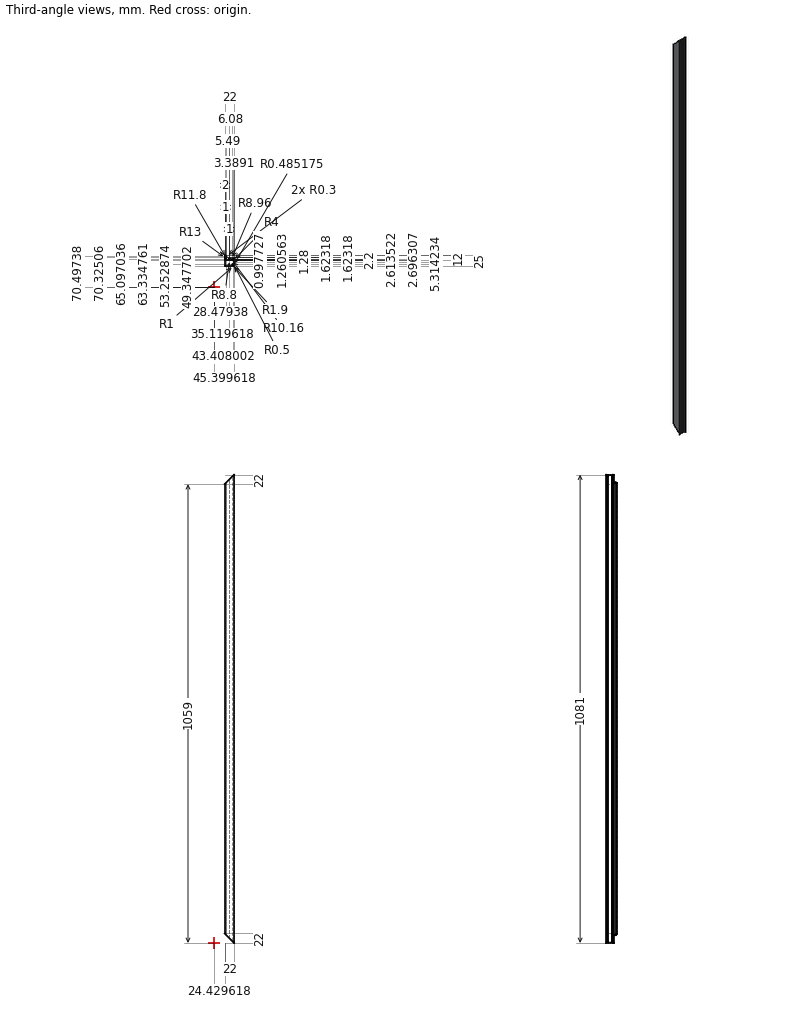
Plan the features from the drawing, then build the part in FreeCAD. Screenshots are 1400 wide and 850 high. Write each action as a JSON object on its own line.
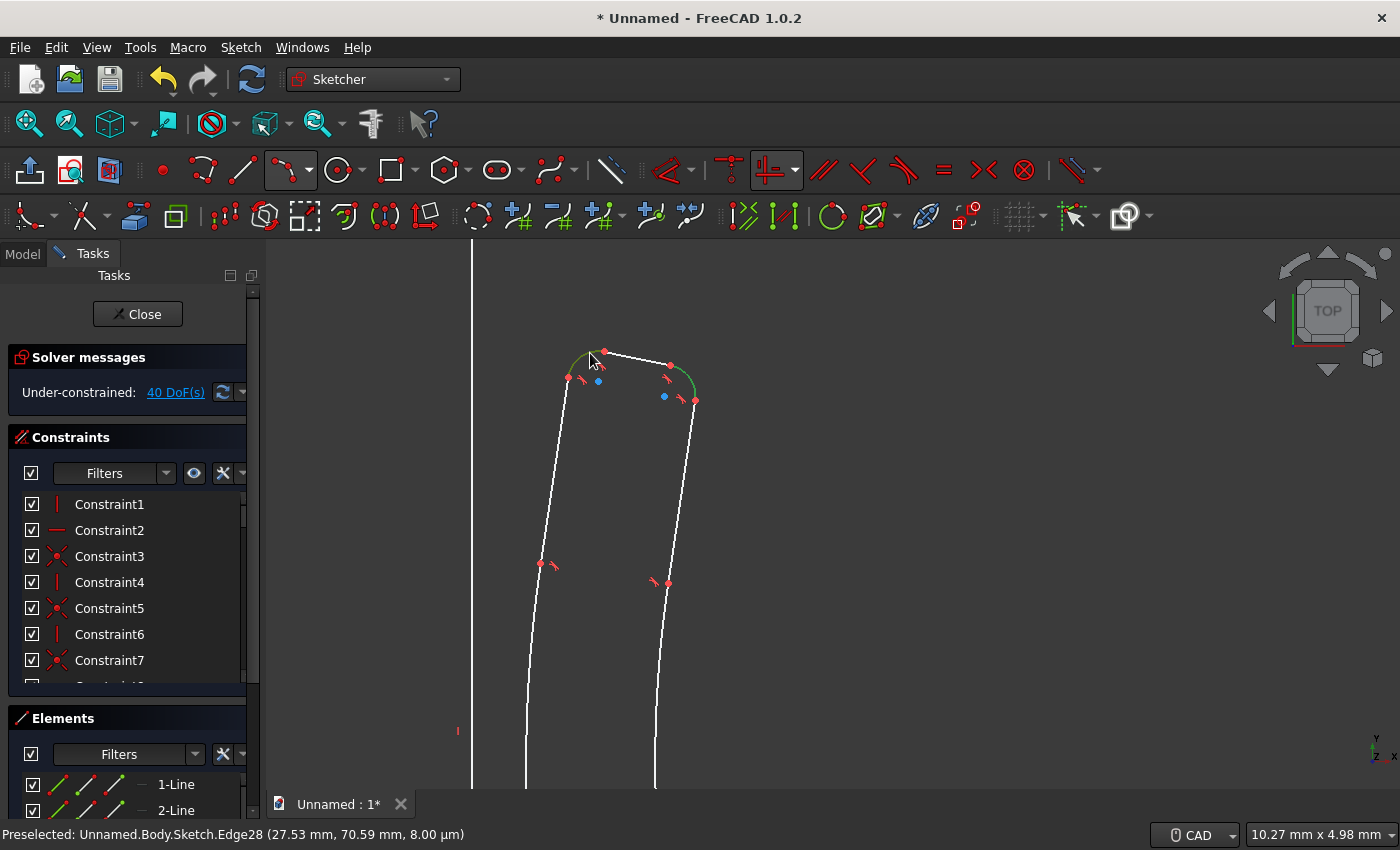
{"action": "left_click", "coordinate": [944, 170]}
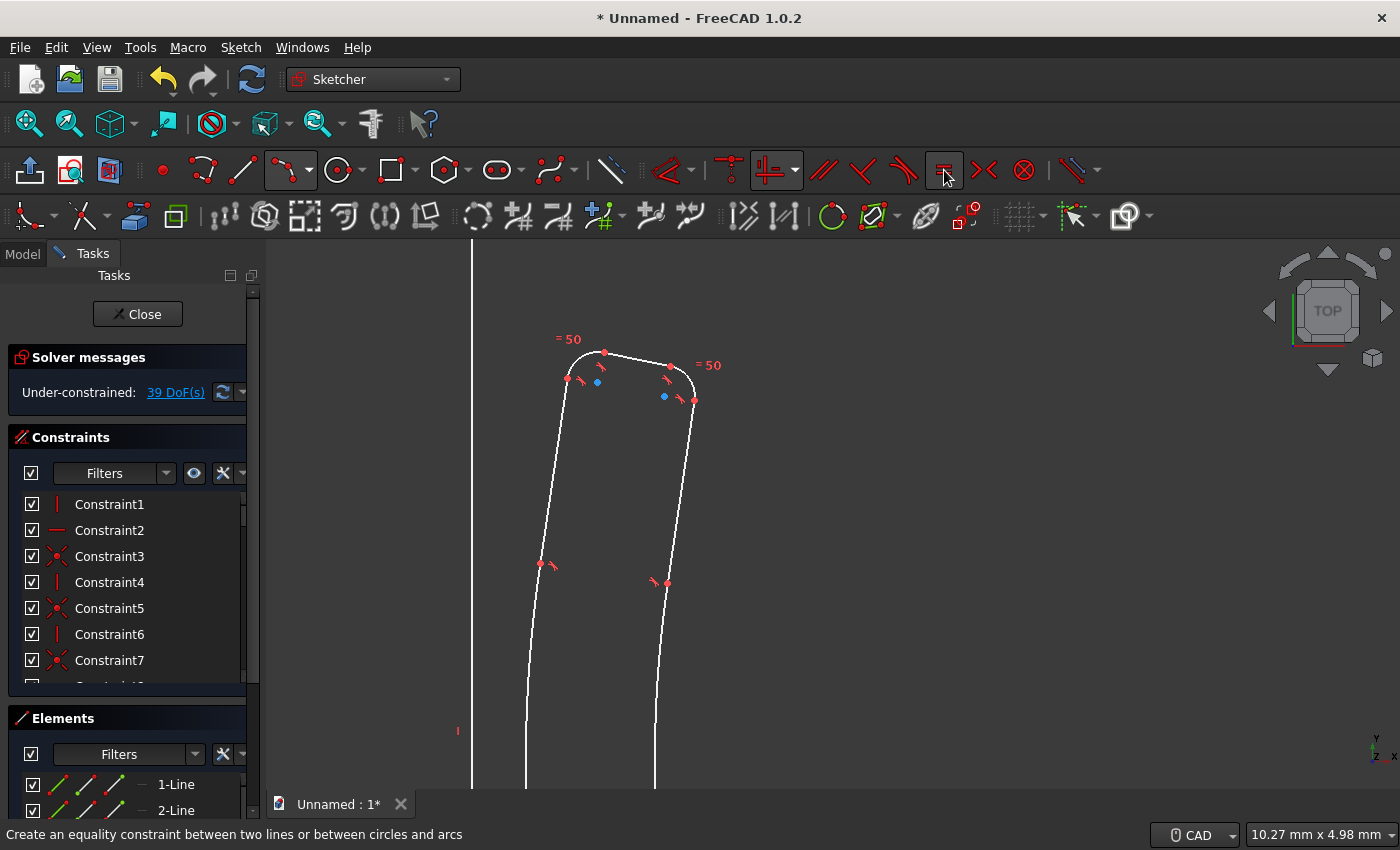
{"action": "scroll", "coordinate": [655, 368], "scroll_direction": "down", "scroll_amount": 10}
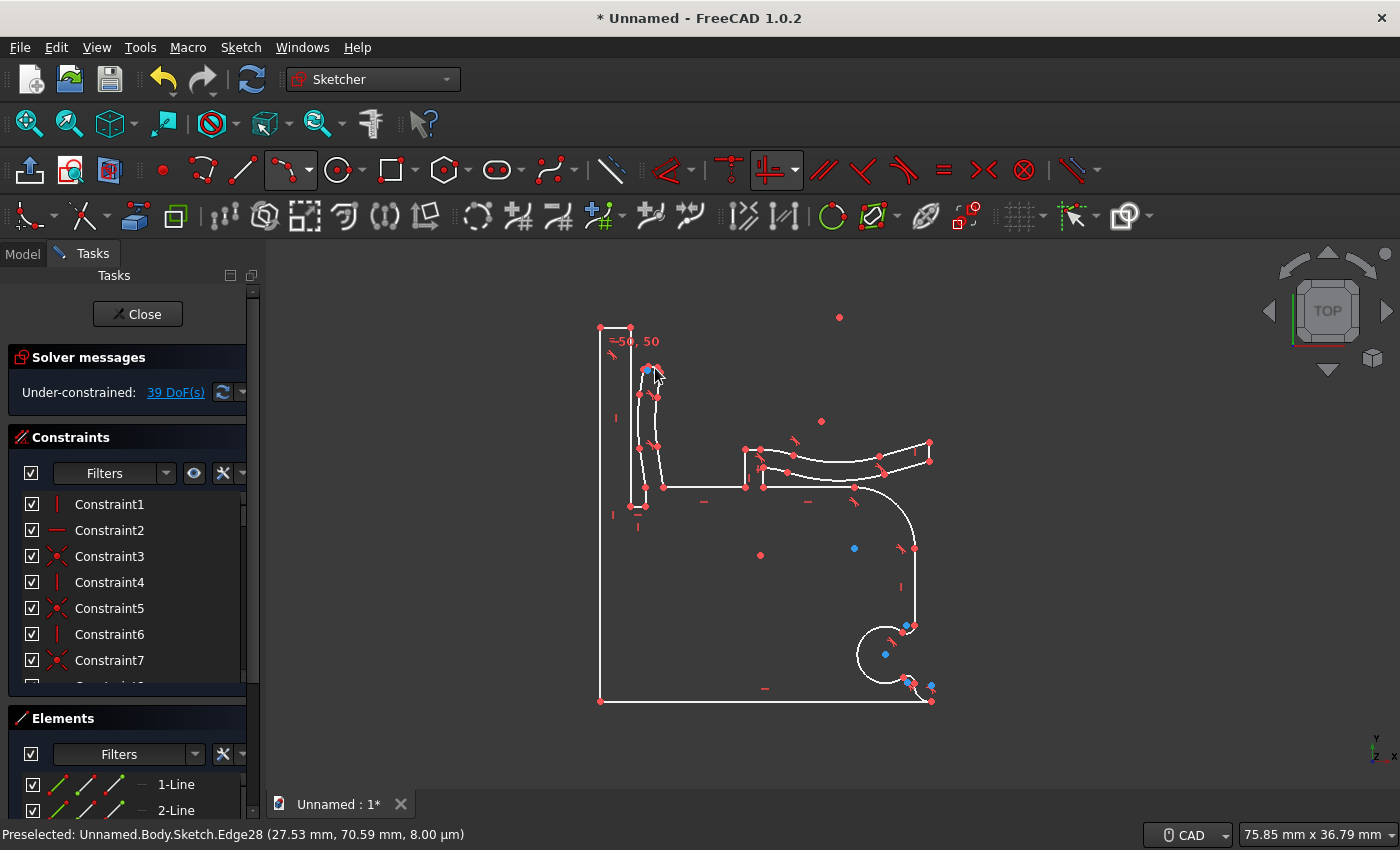
{"action": "left_click", "coordinate": [908, 521]}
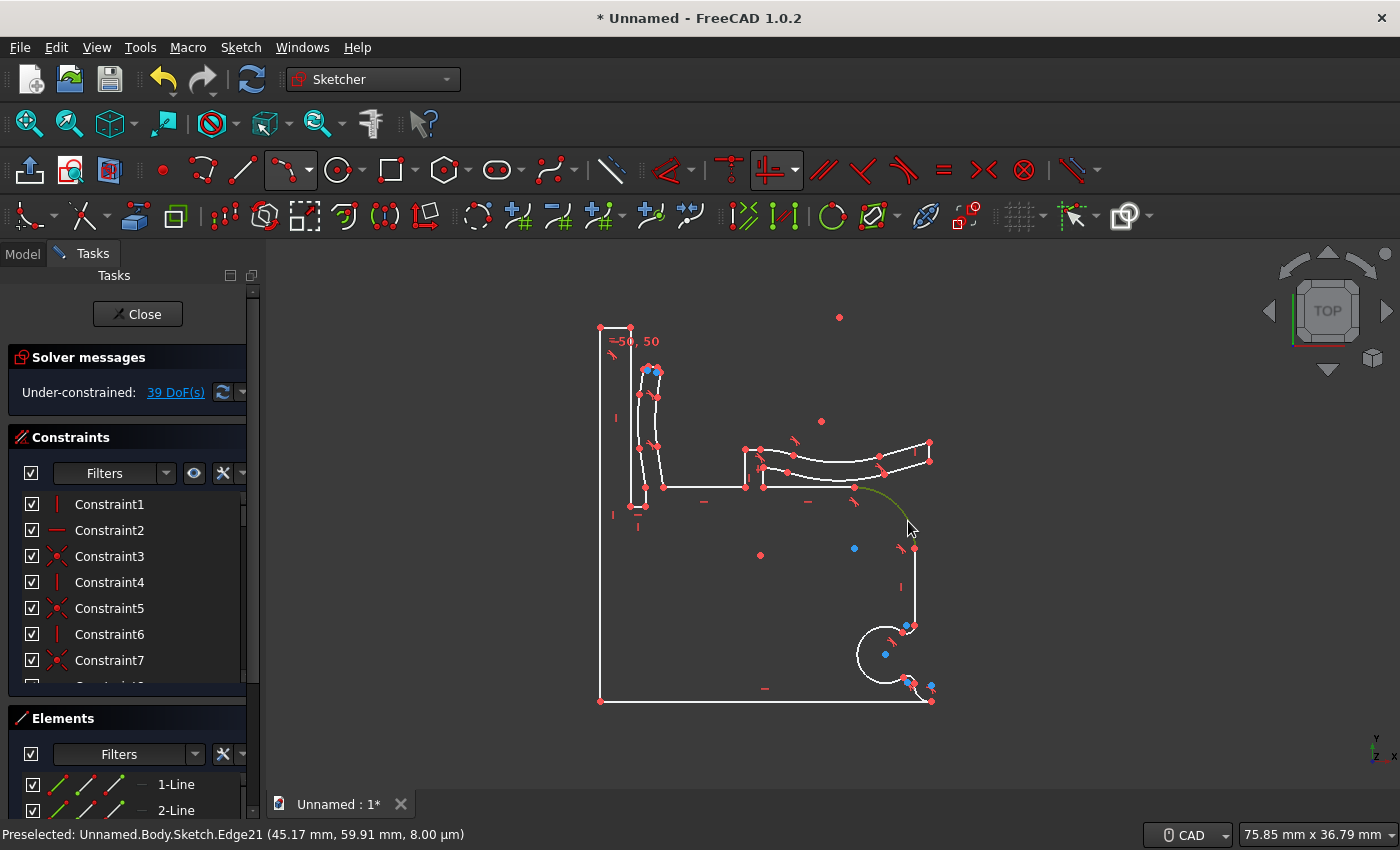
{"action": "key", "text": "k r"}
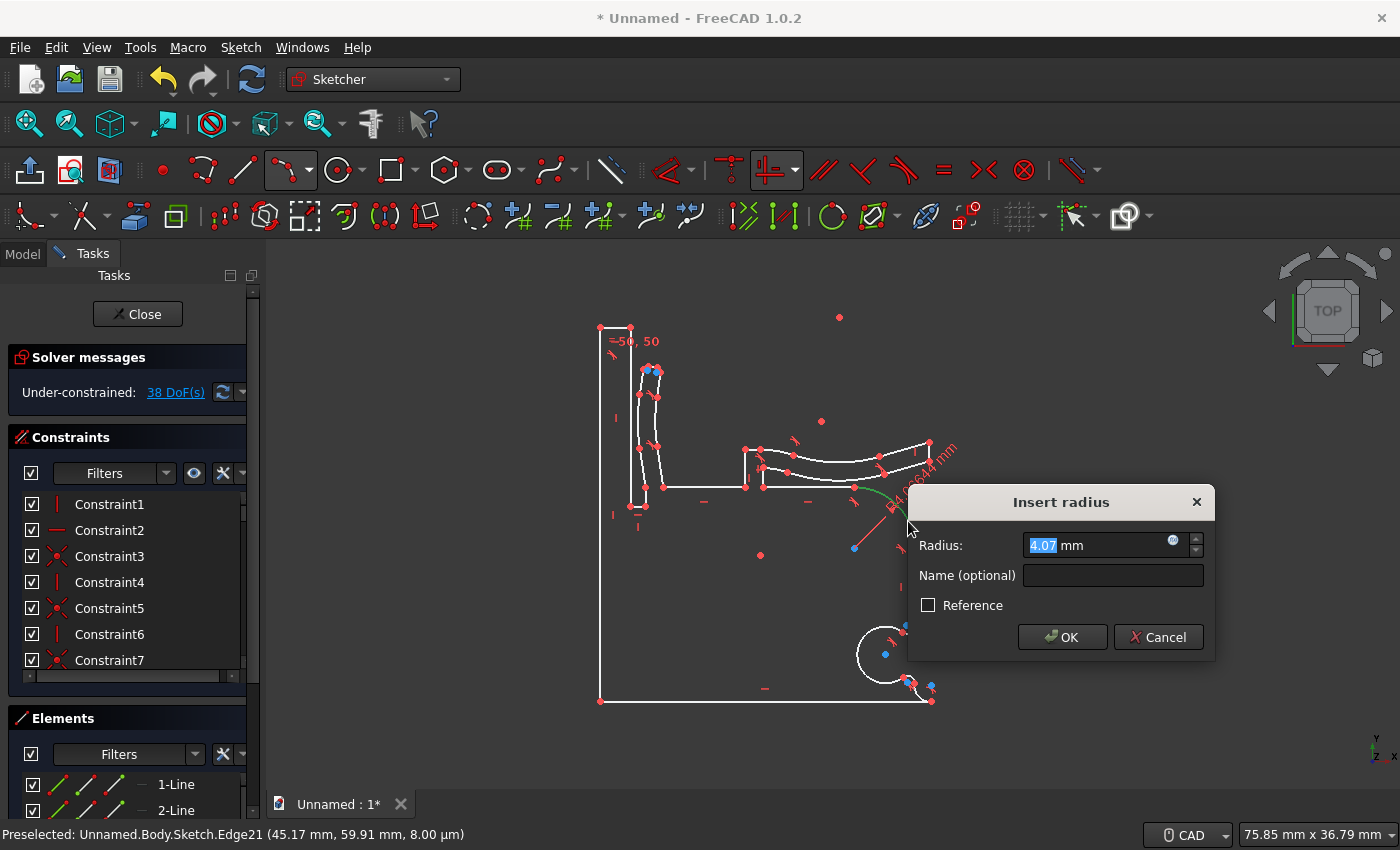
{"action": "type", "text": "4"}
{"action": "key", "text": "Return"}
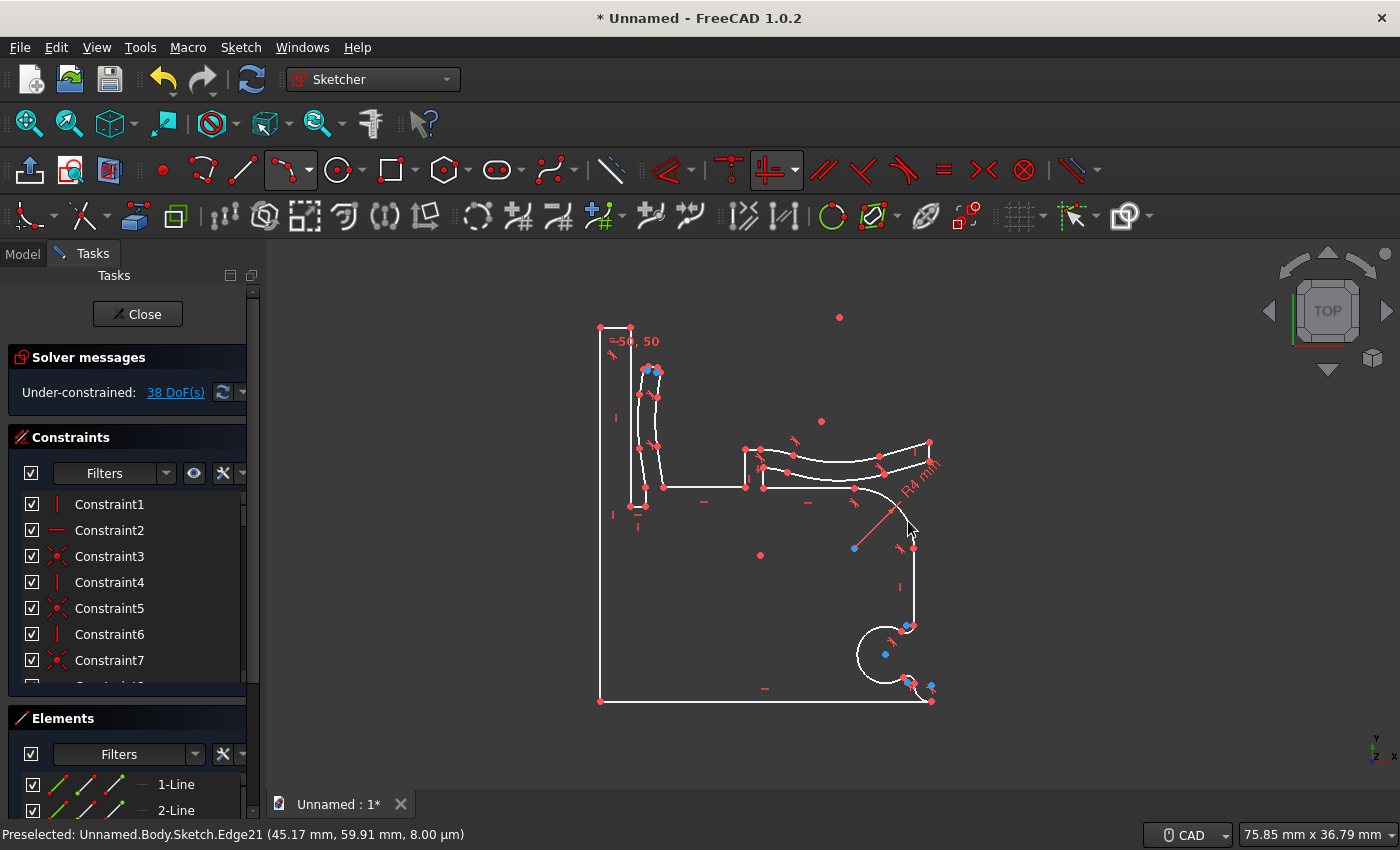
{"action": "left_click", "coordinate": [776, 469]}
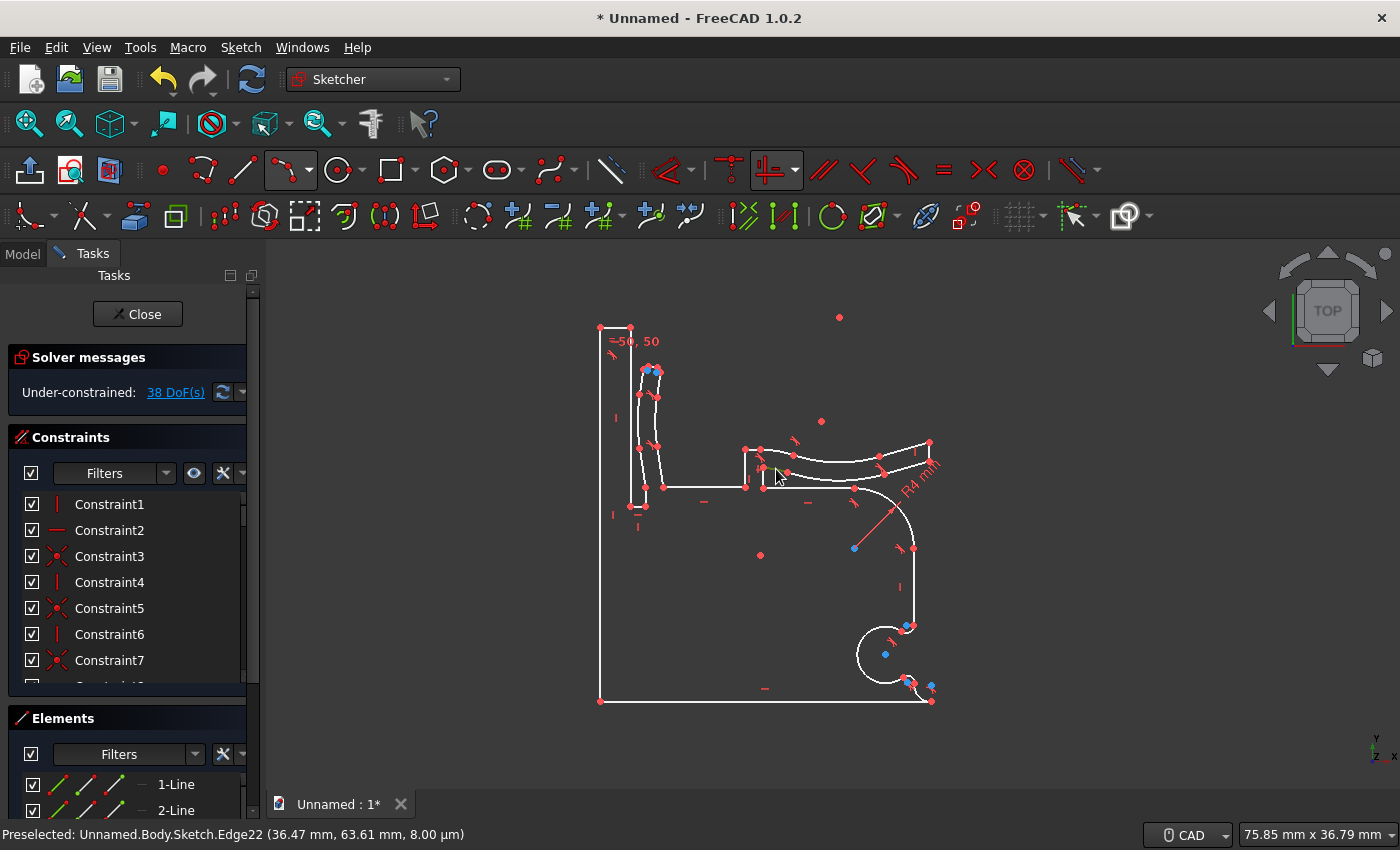
{"action": "key", "text": "k r"}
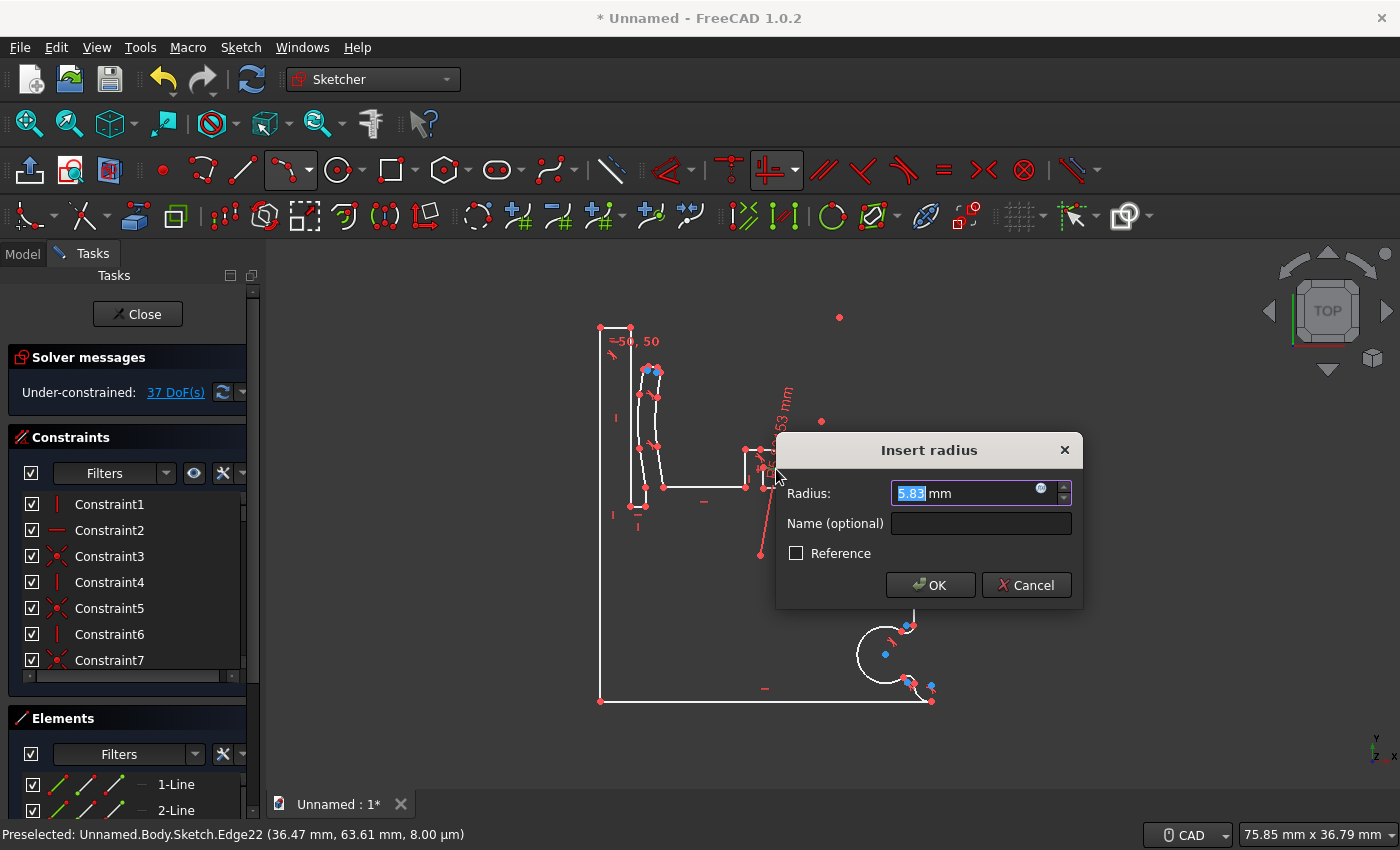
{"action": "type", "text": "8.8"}
{"action": "key", "text": "Return"}